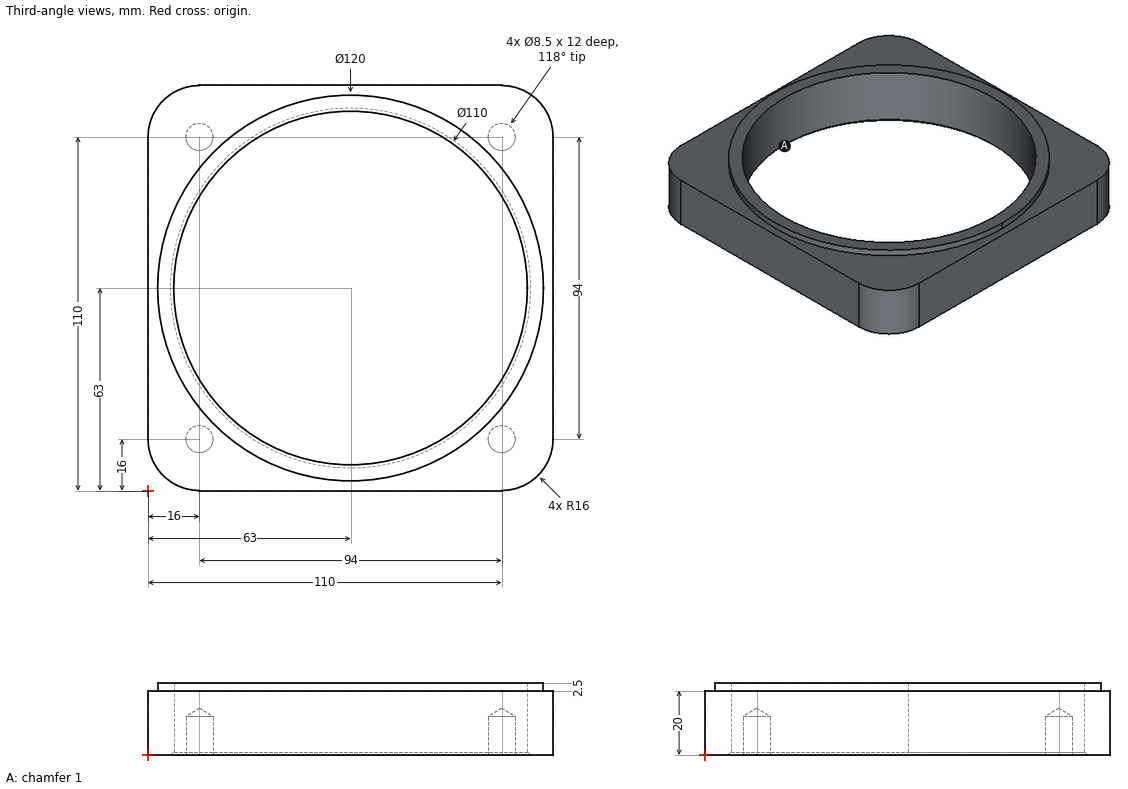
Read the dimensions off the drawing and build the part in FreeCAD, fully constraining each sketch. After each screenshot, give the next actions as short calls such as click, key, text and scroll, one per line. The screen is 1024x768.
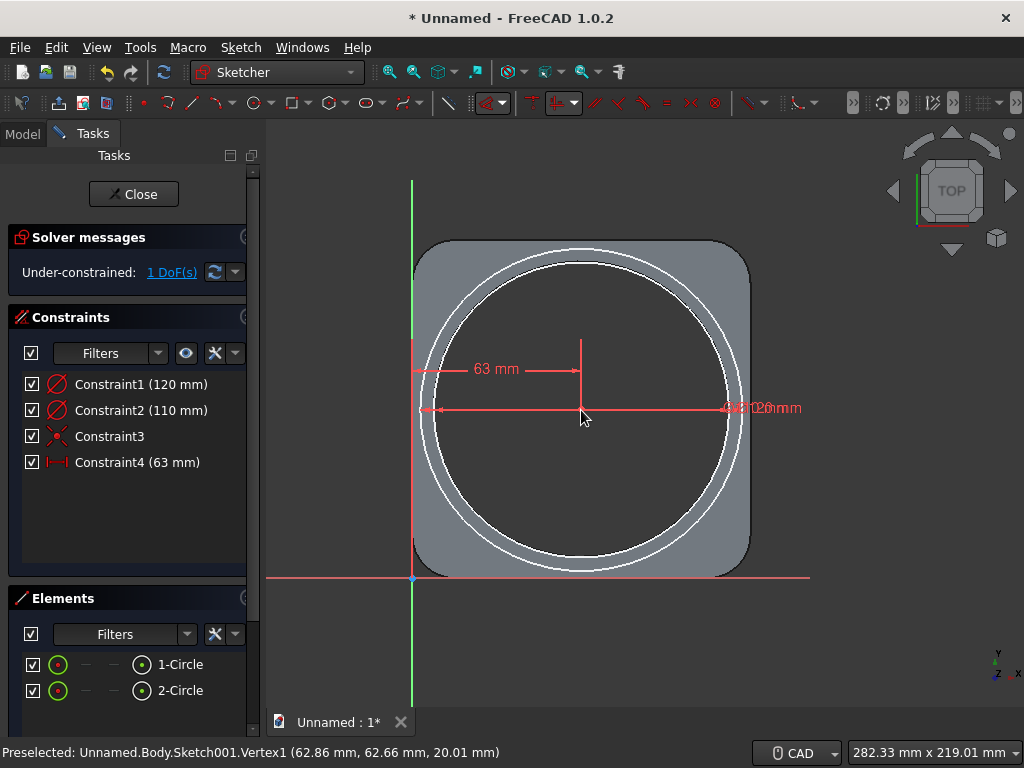
click(581, 410)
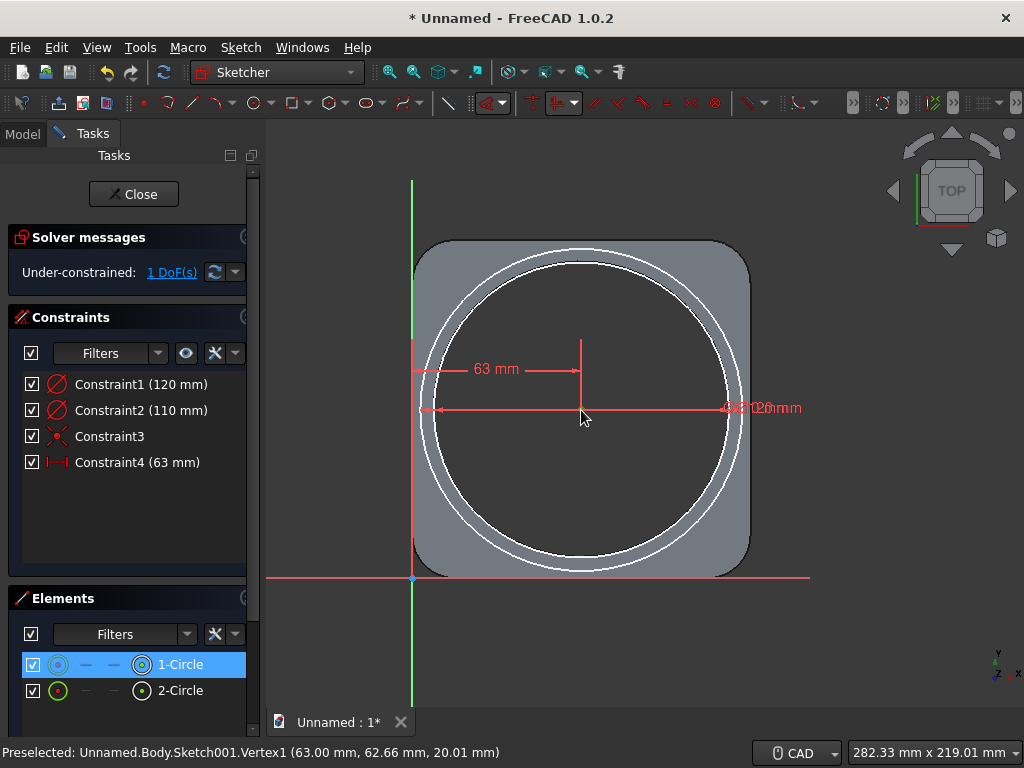
click(504, 104)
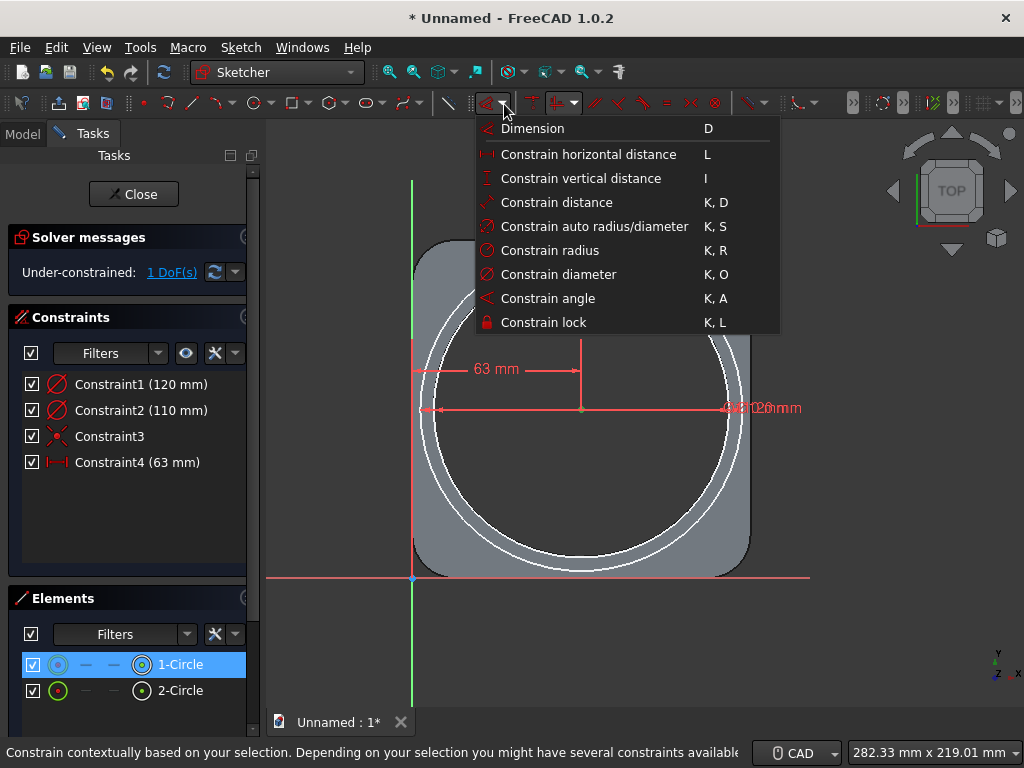
click(628, 178)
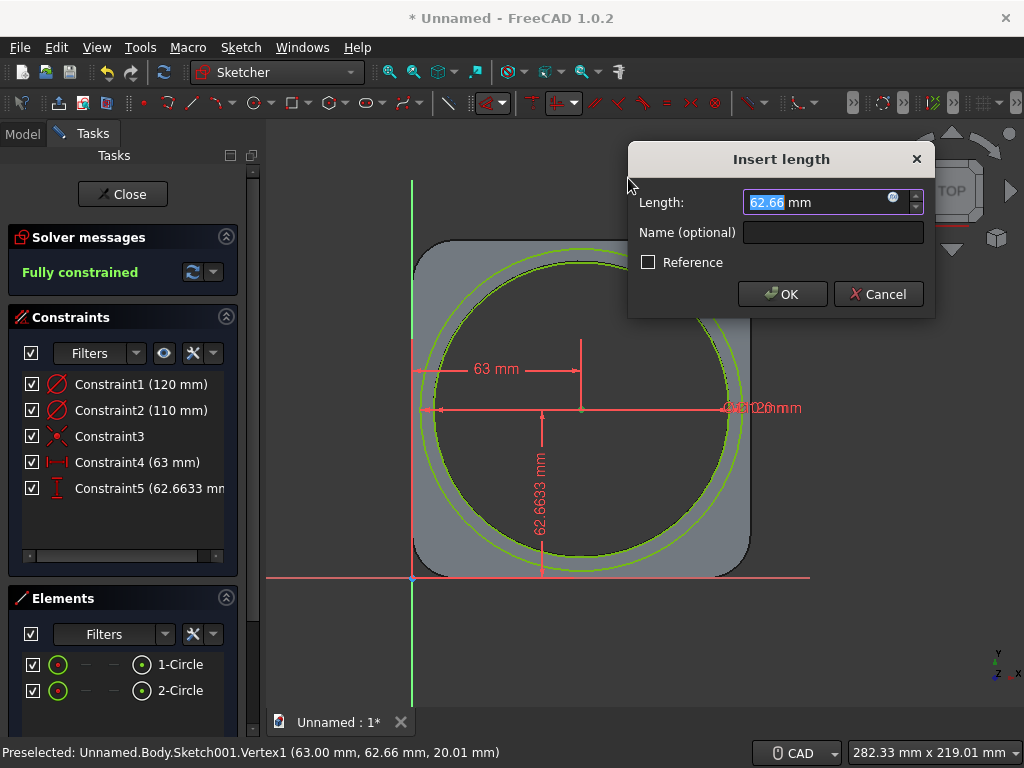
text(63)
key(Return)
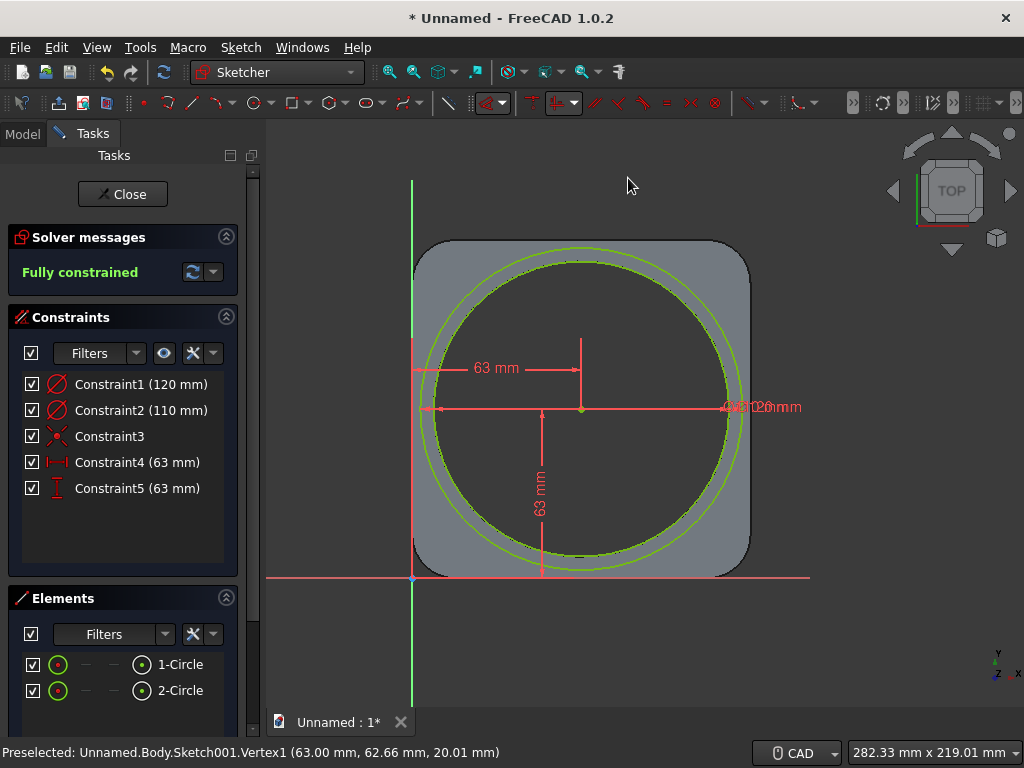
click(123, 194)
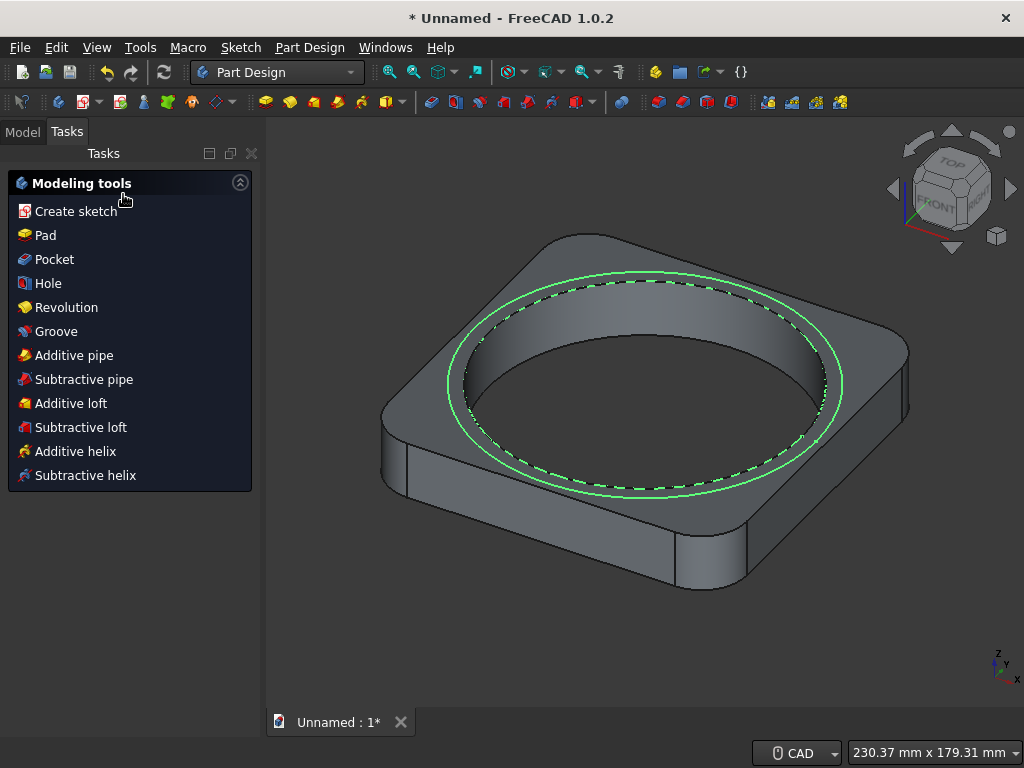
click(266, 102)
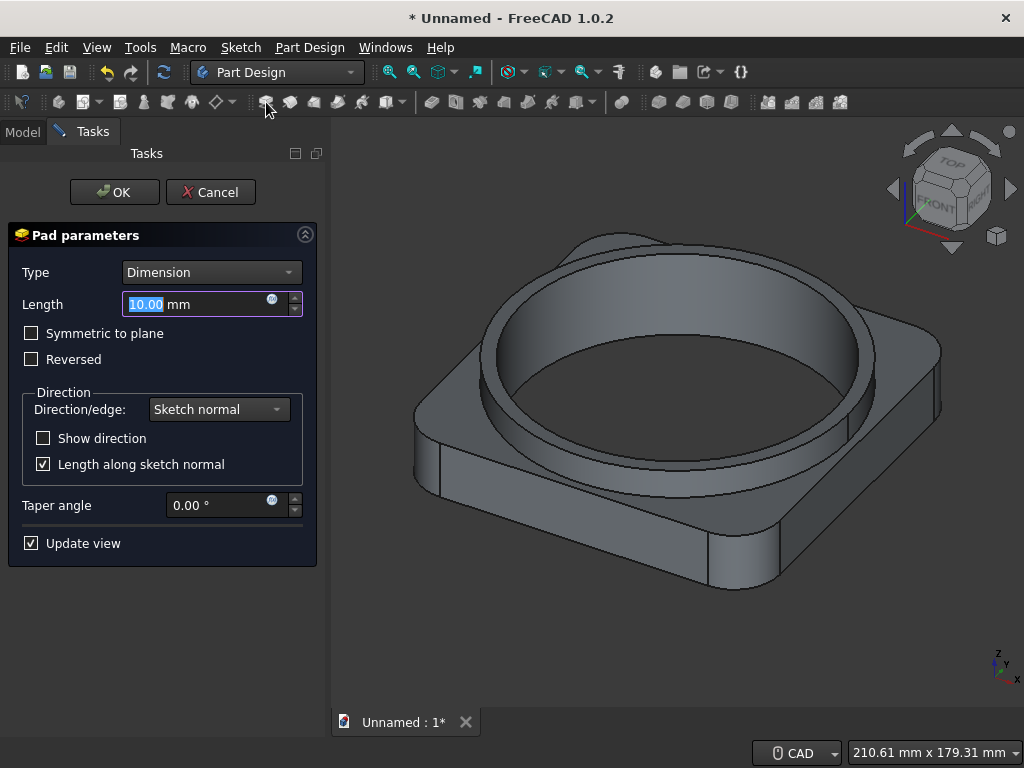
text(2.5)
key(Tab)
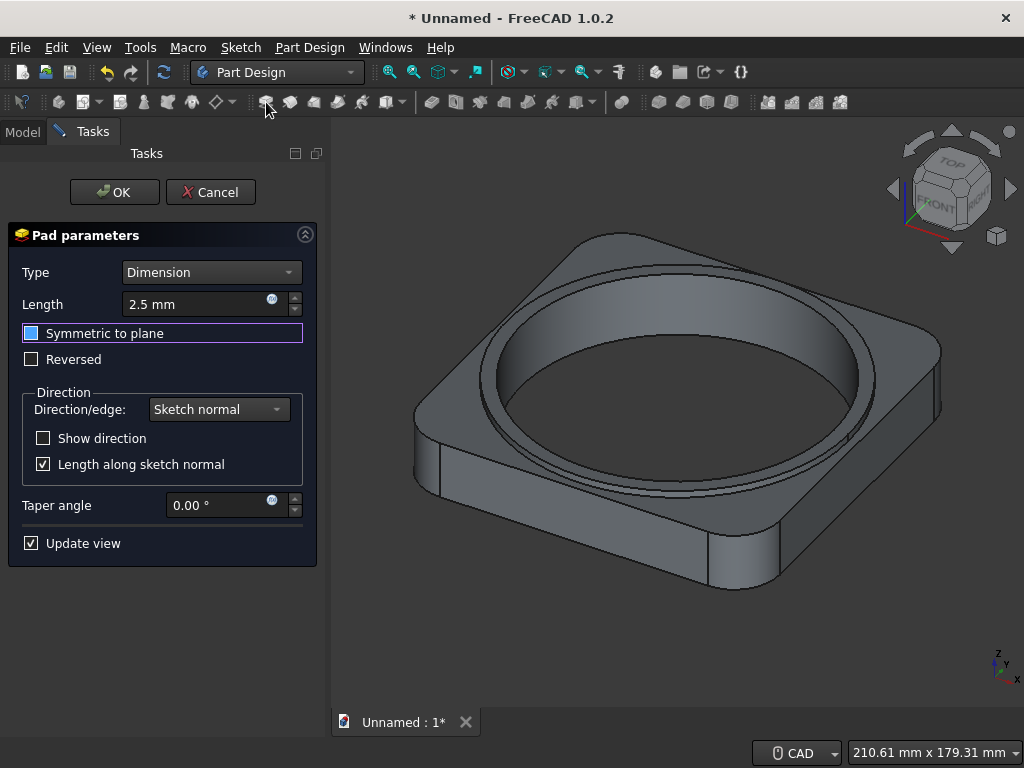
click(115, 192)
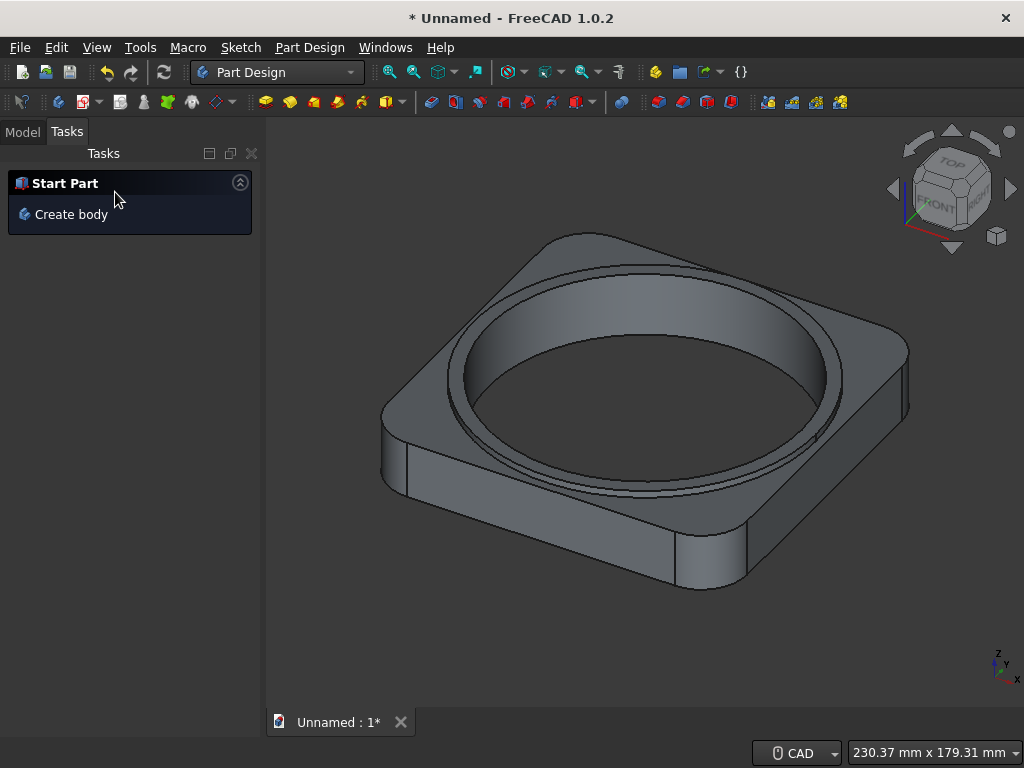
click(84, 102)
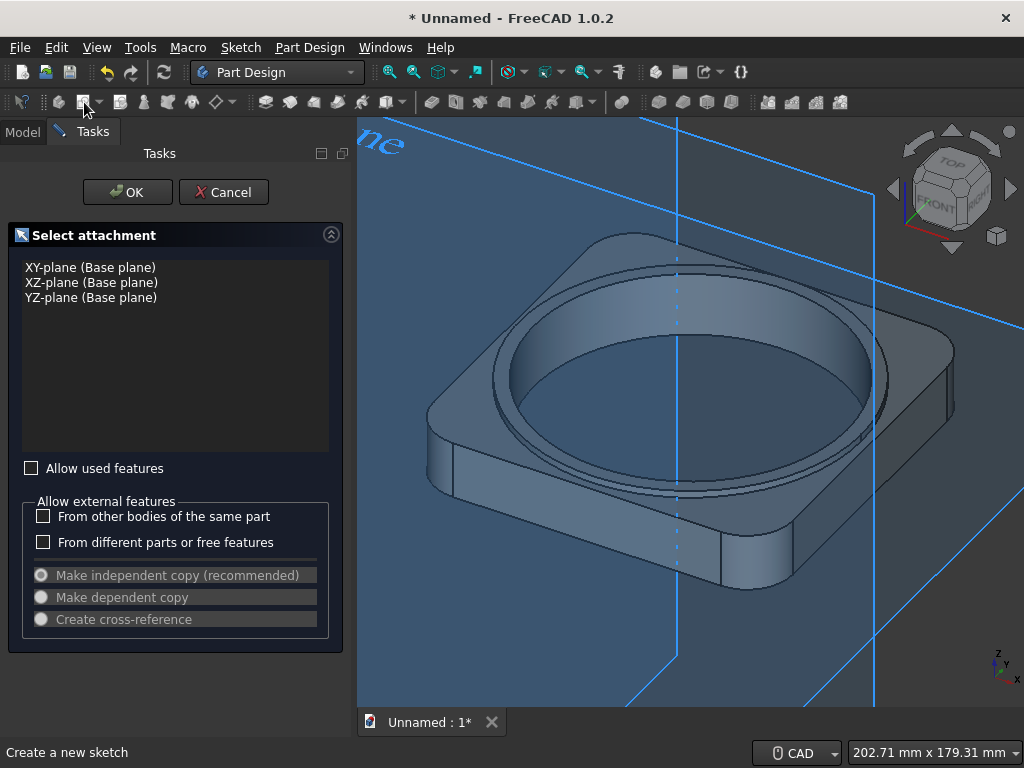
click(82, 268)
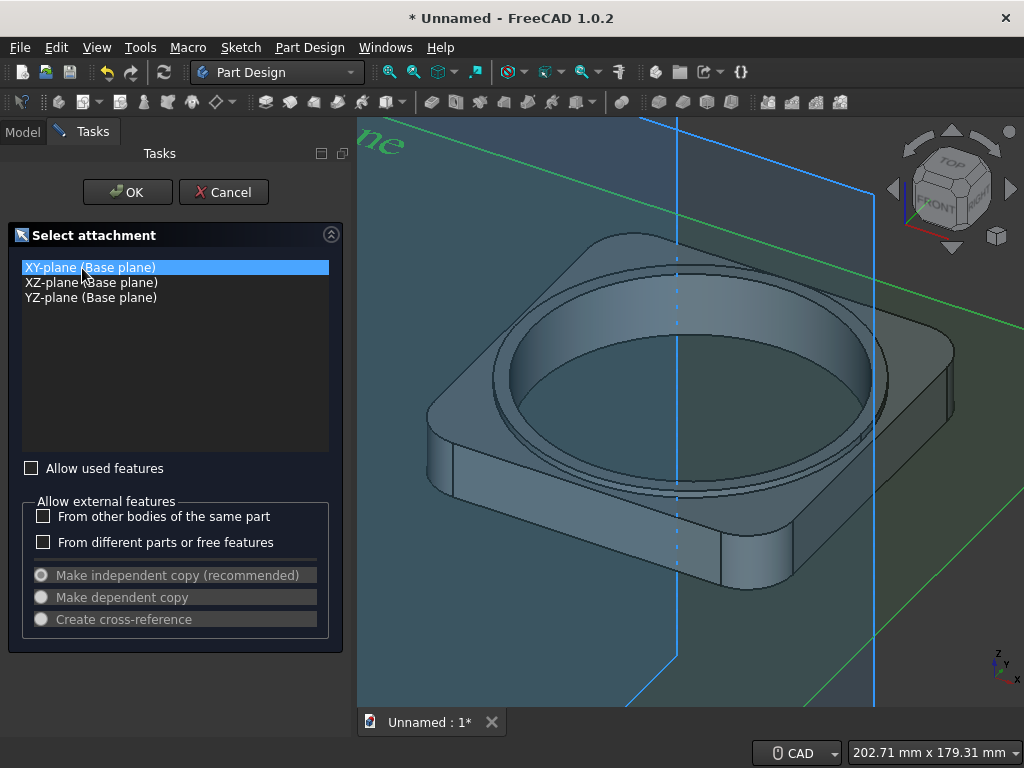
click(128, 192)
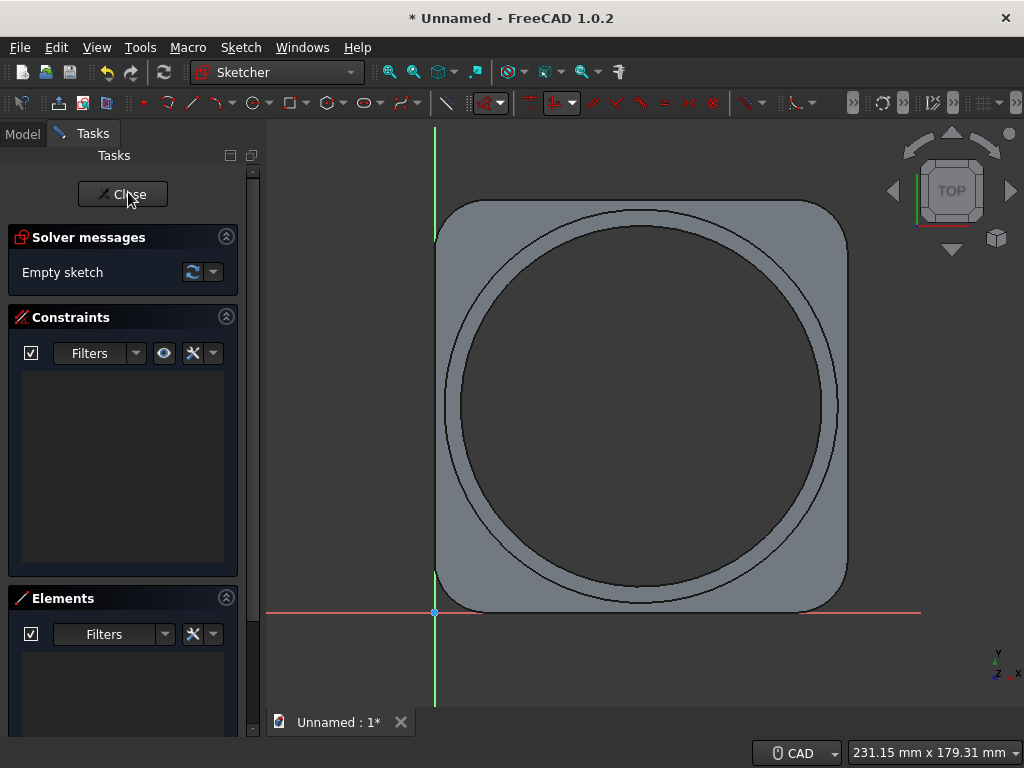
click(108, 104)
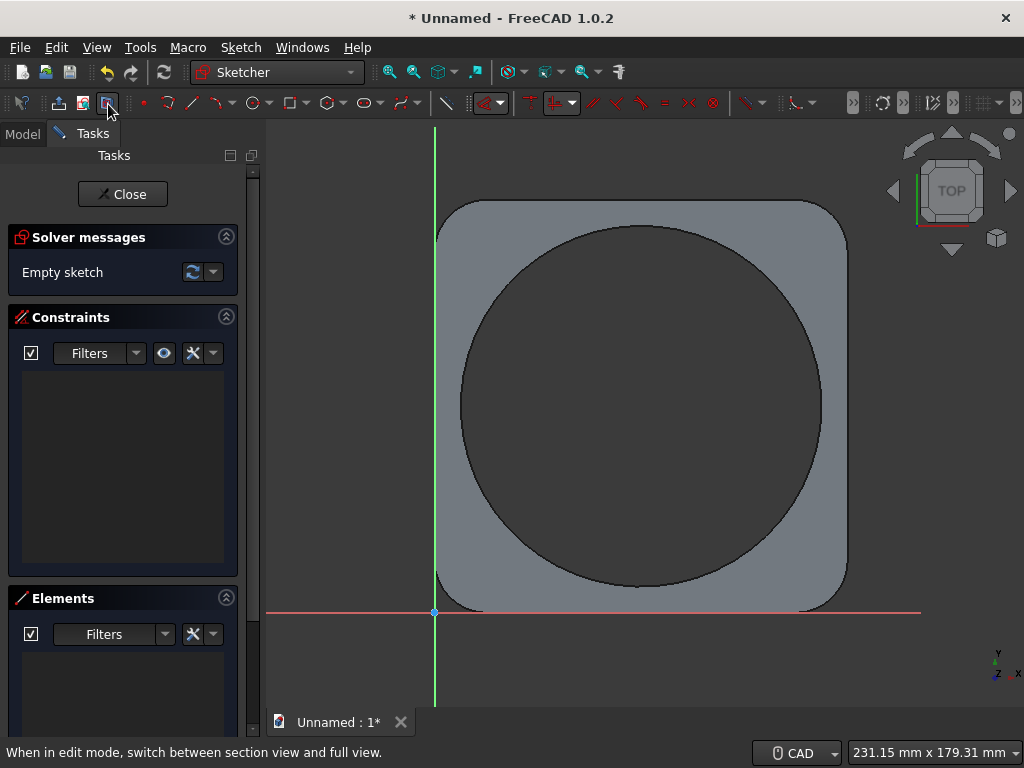
click(254, 104)